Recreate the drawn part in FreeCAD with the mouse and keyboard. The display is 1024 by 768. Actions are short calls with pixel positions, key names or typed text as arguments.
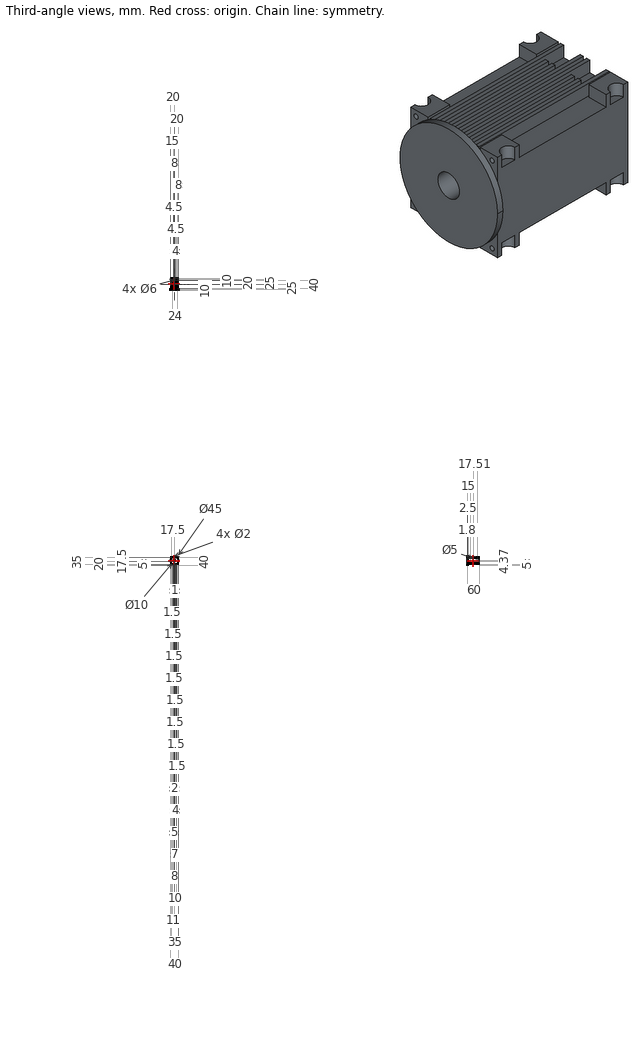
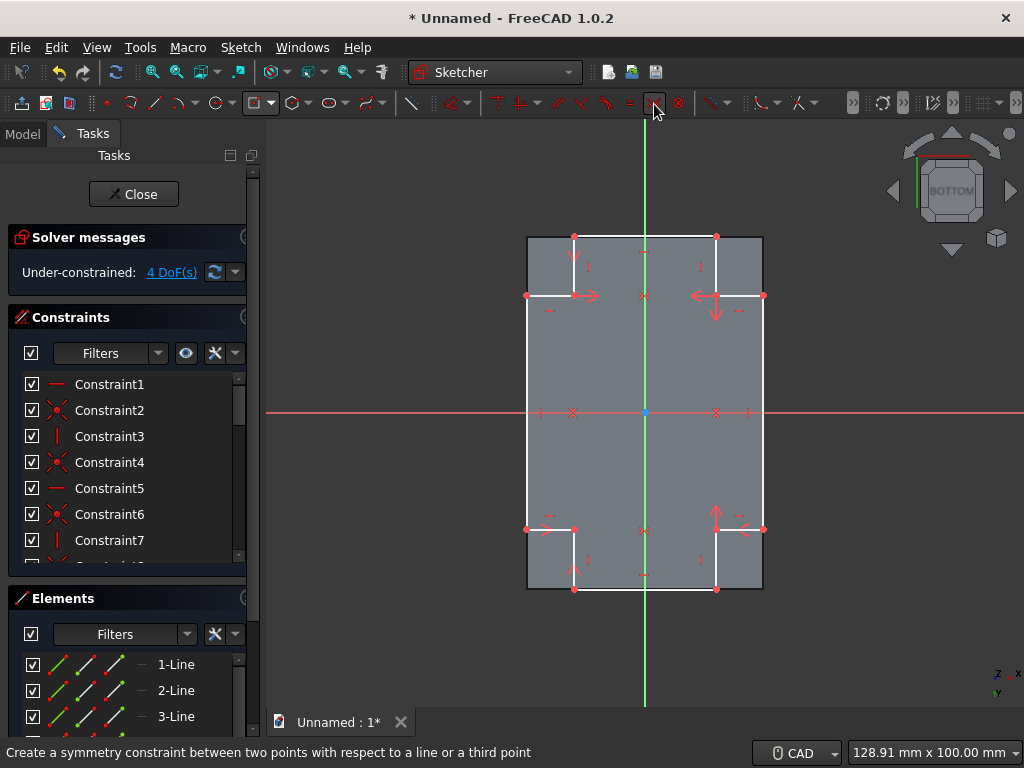
click(450, 104)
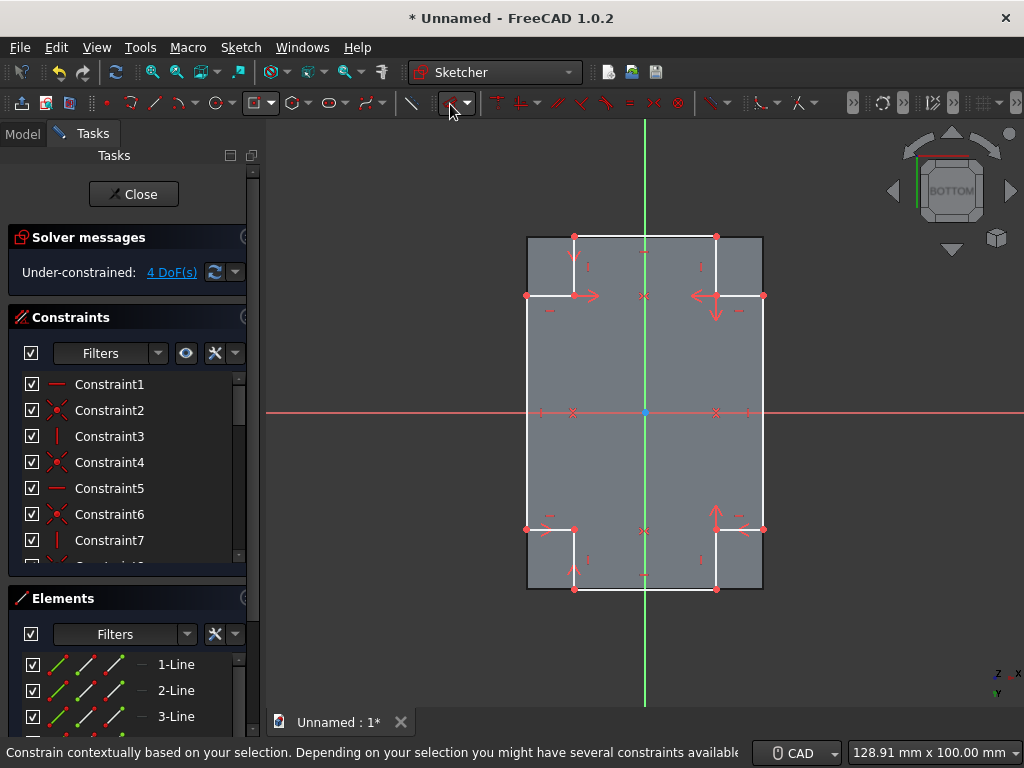
click(730, 530)
click(740, 564)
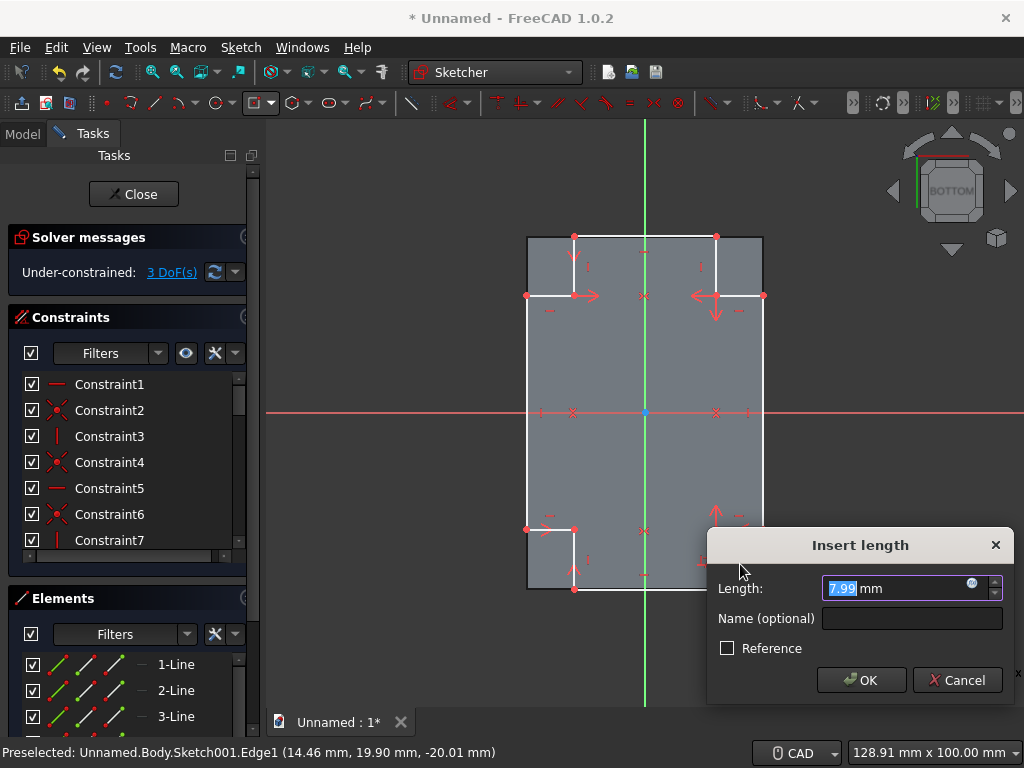
text(8)
key(Return)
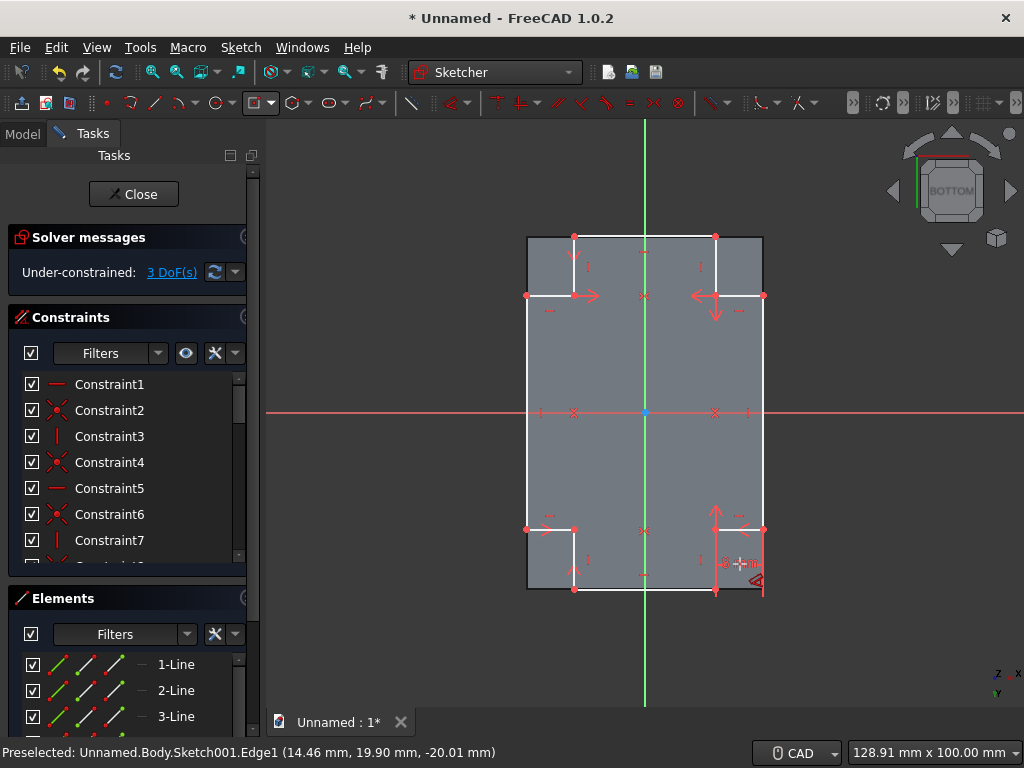
click(763, 460)
click(797, 359)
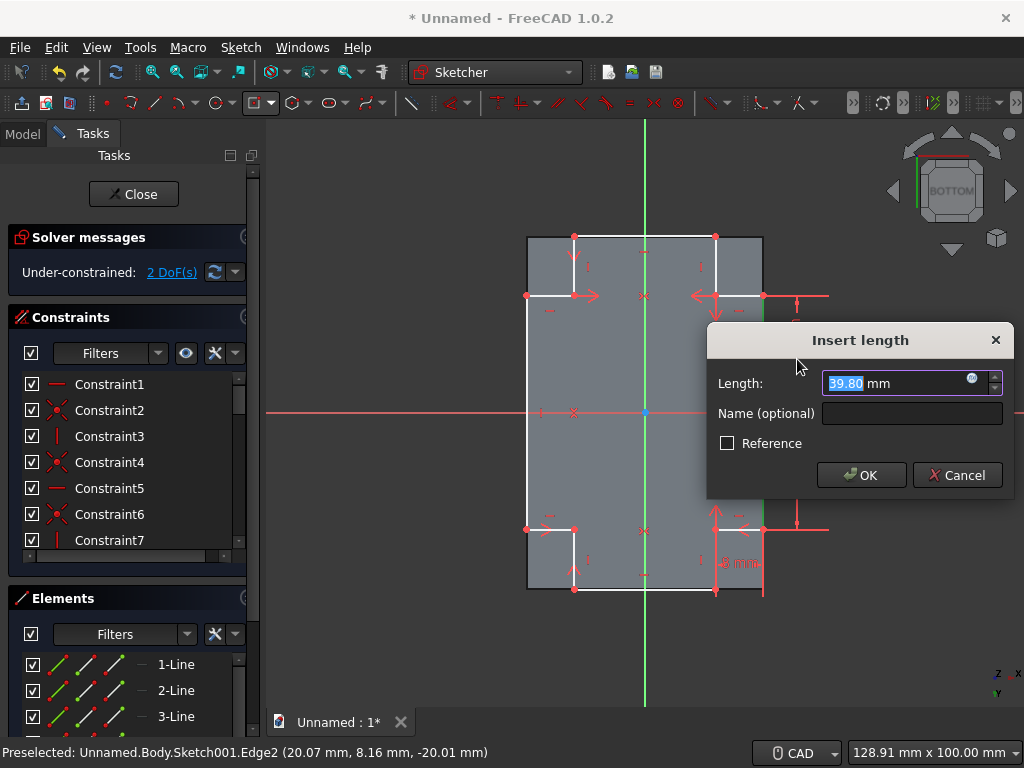
text(40)
key(Return)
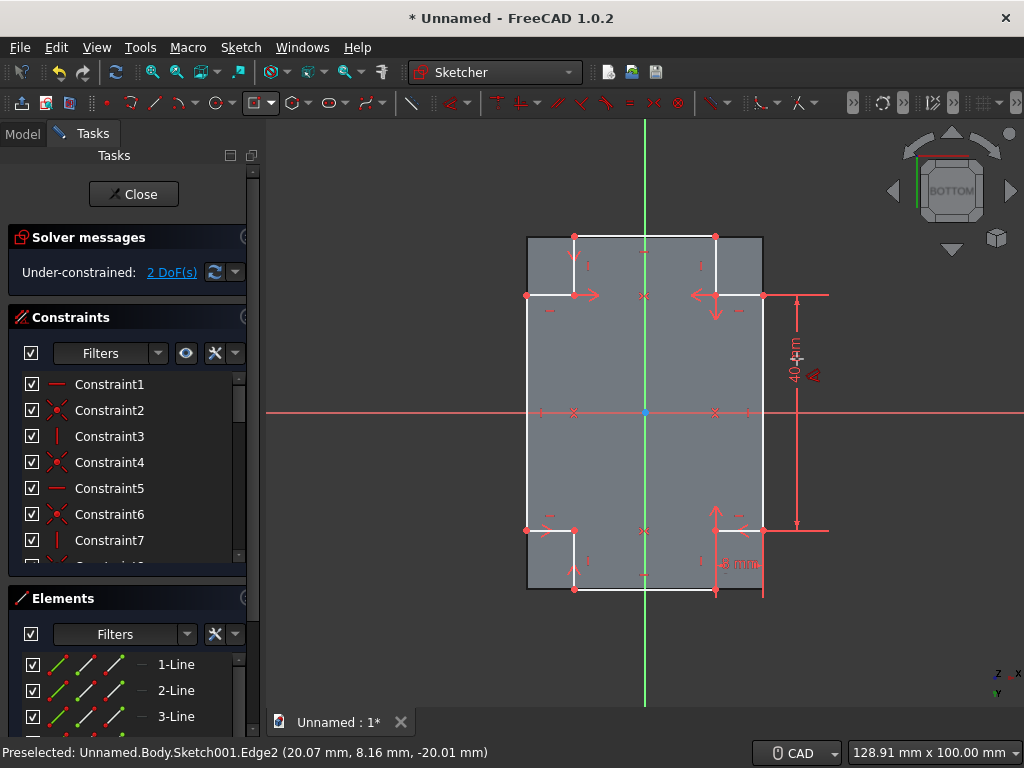
click(716, 278)
click(750, 266)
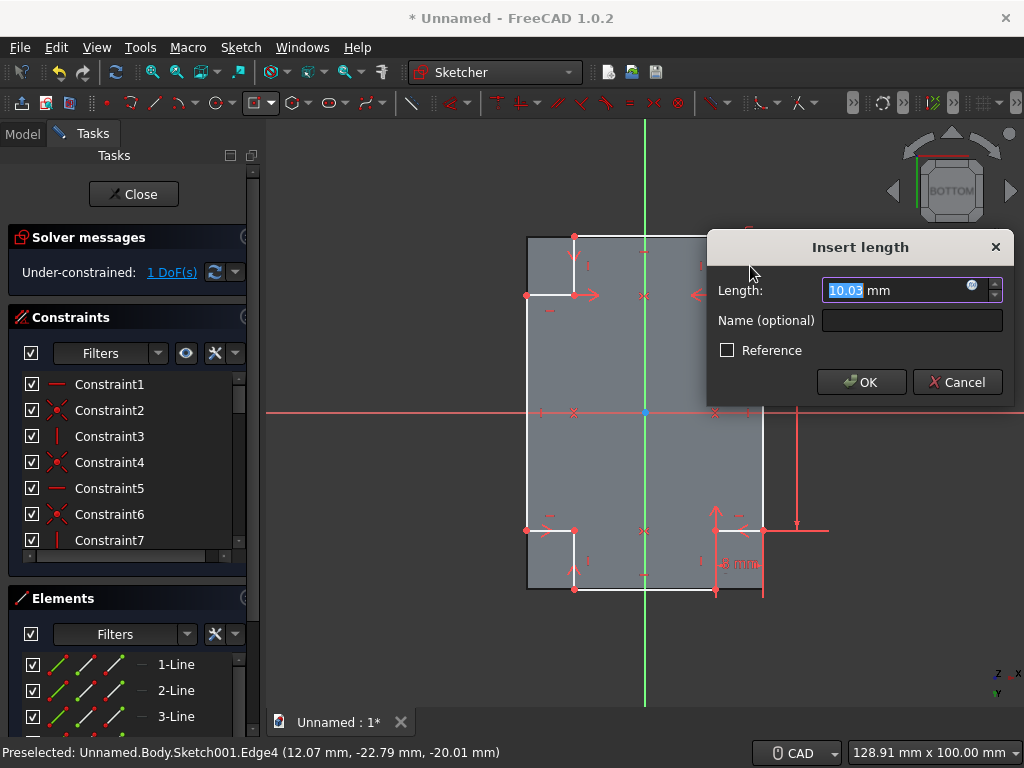
text(10)
key(Return)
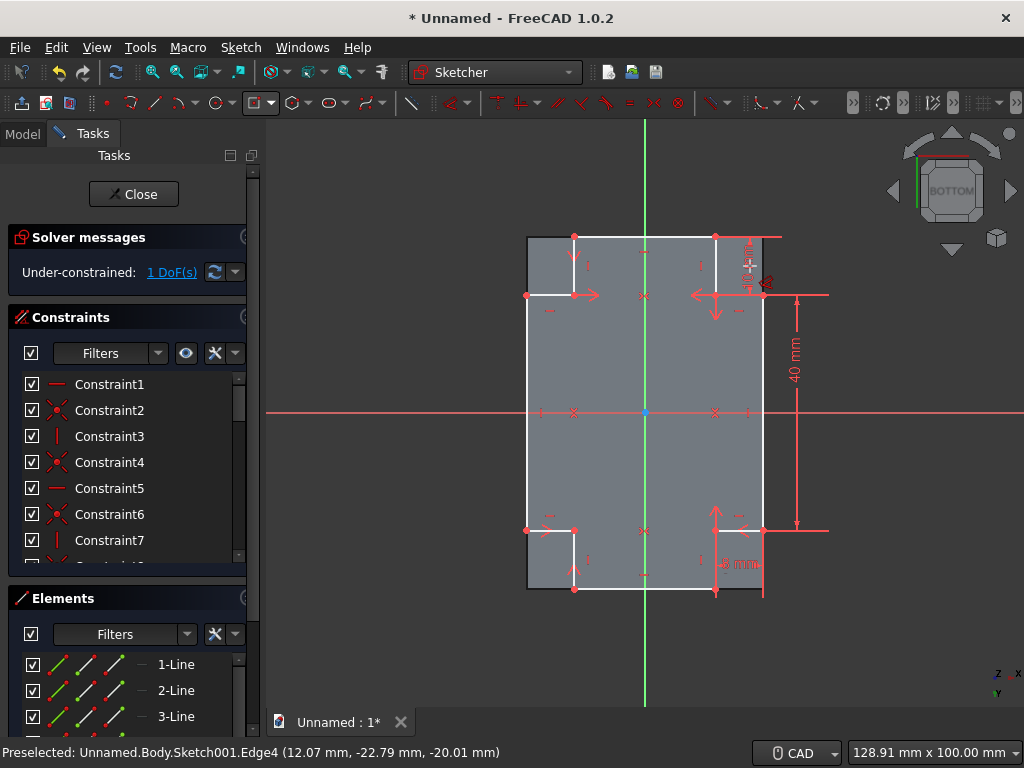
click(673, 237)
click(612, 203)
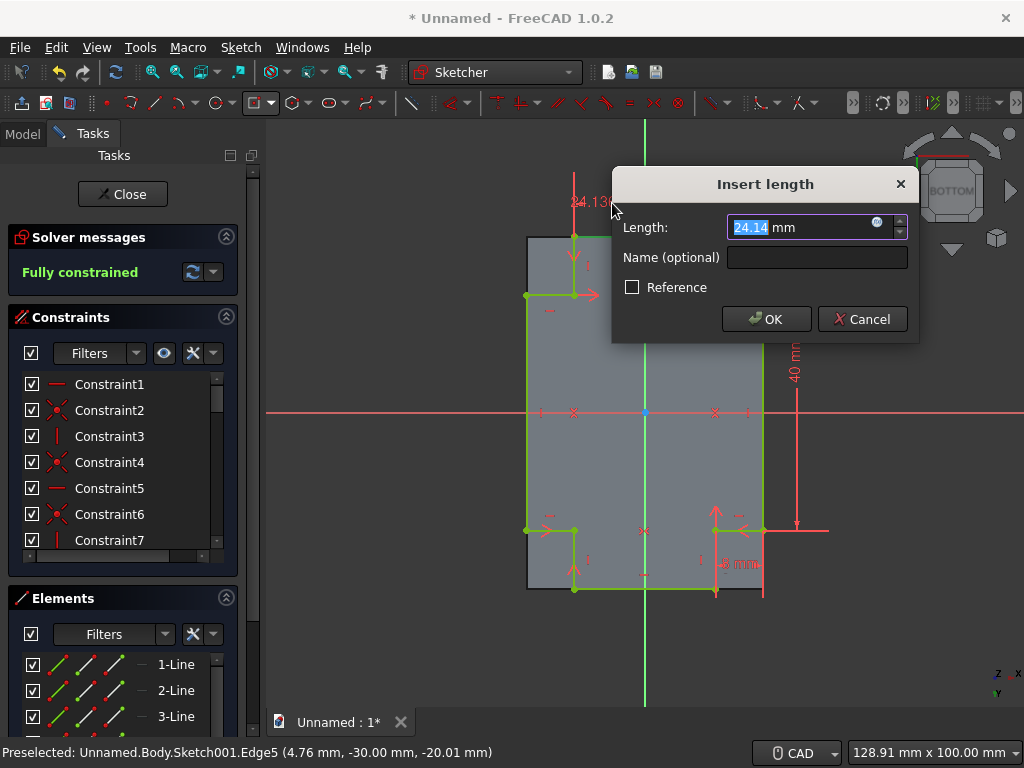
text(24)
key(Return)
key(Escape)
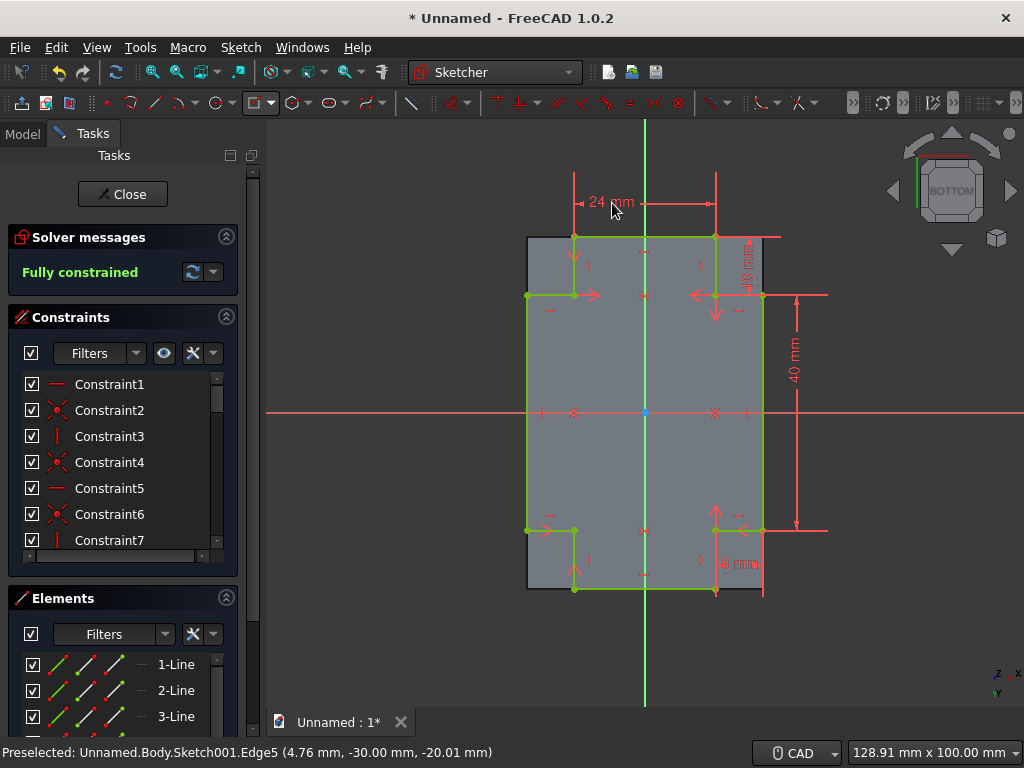
click(123, 194)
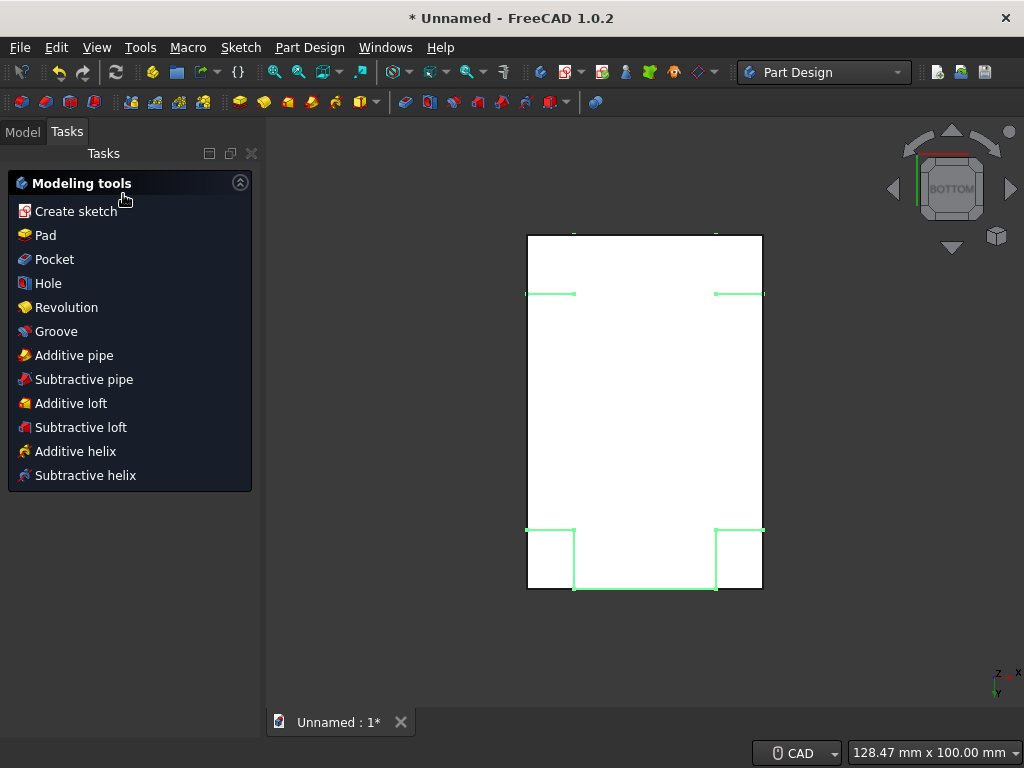
click(406, 102)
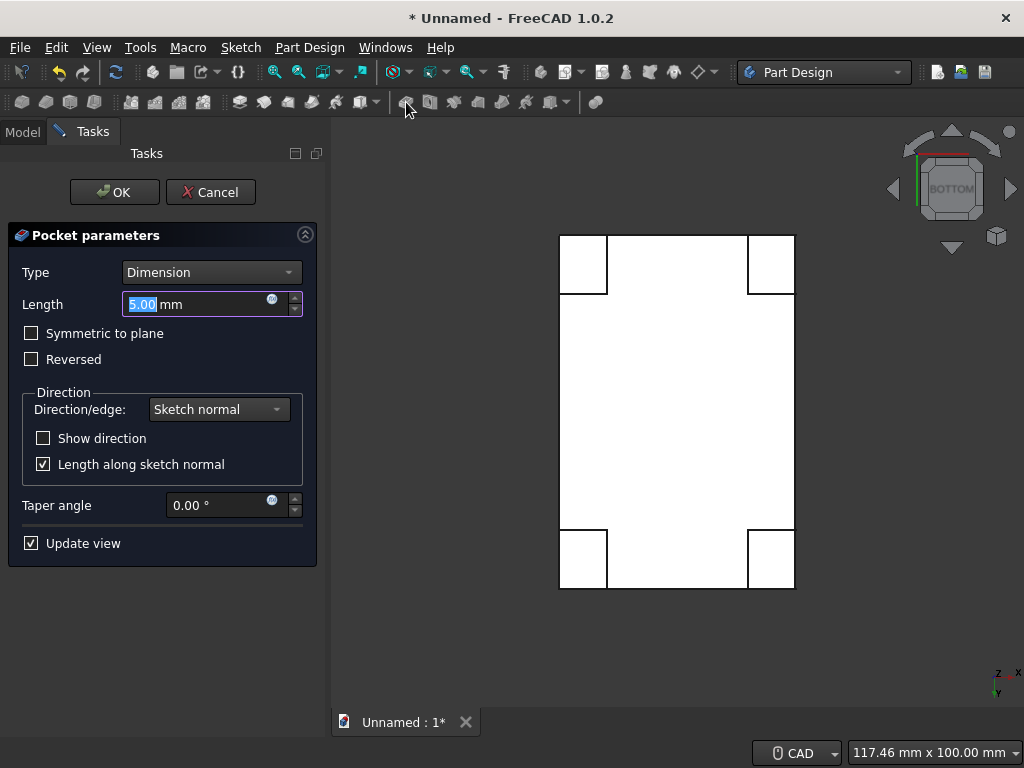
text(5)
key(Tab)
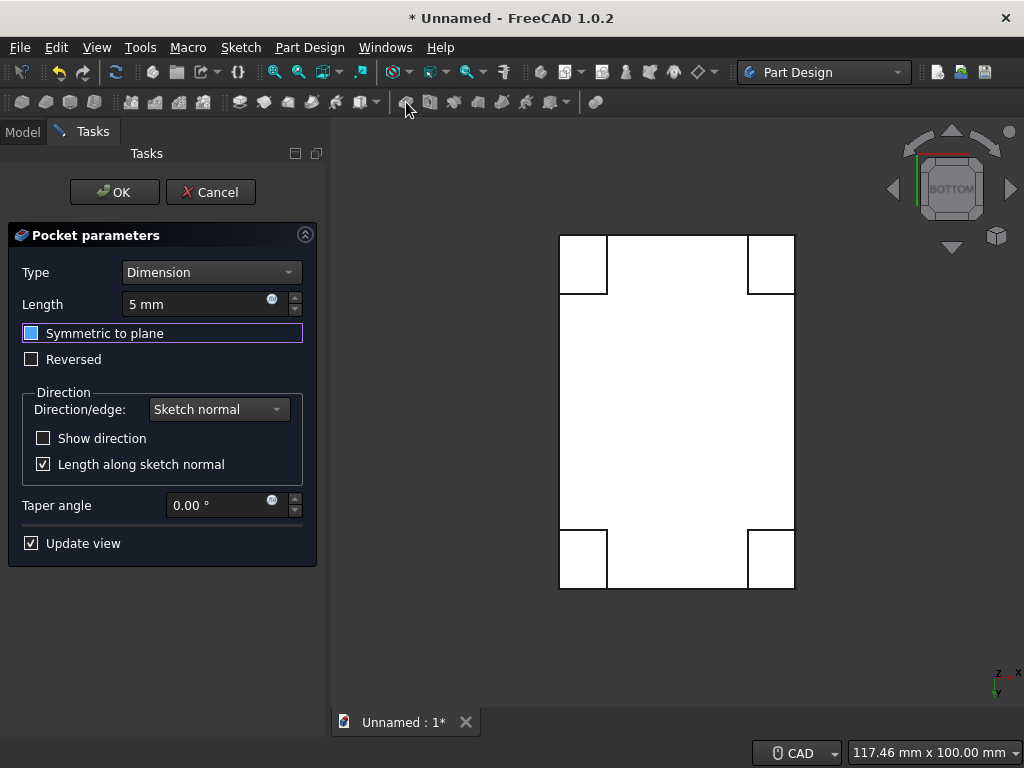
click(115, 192)